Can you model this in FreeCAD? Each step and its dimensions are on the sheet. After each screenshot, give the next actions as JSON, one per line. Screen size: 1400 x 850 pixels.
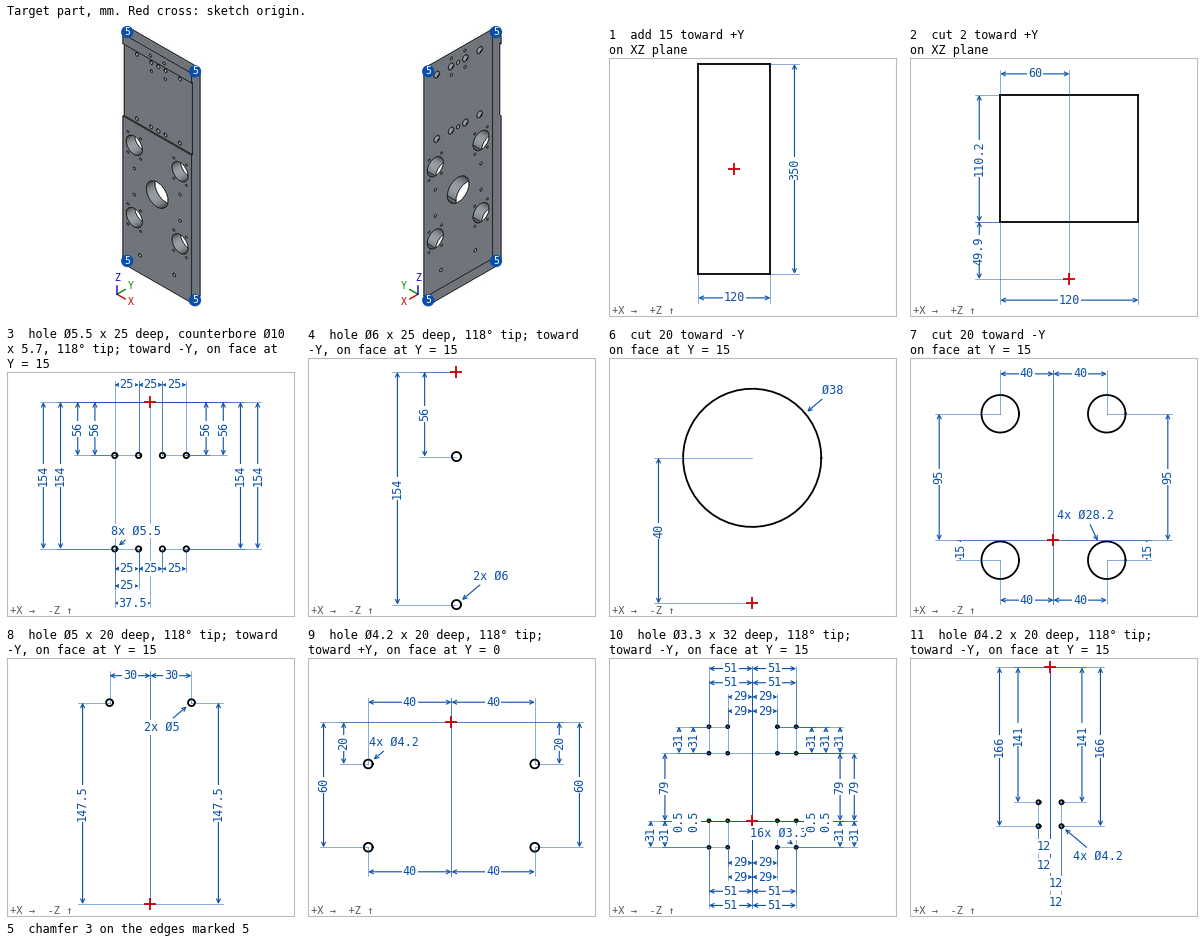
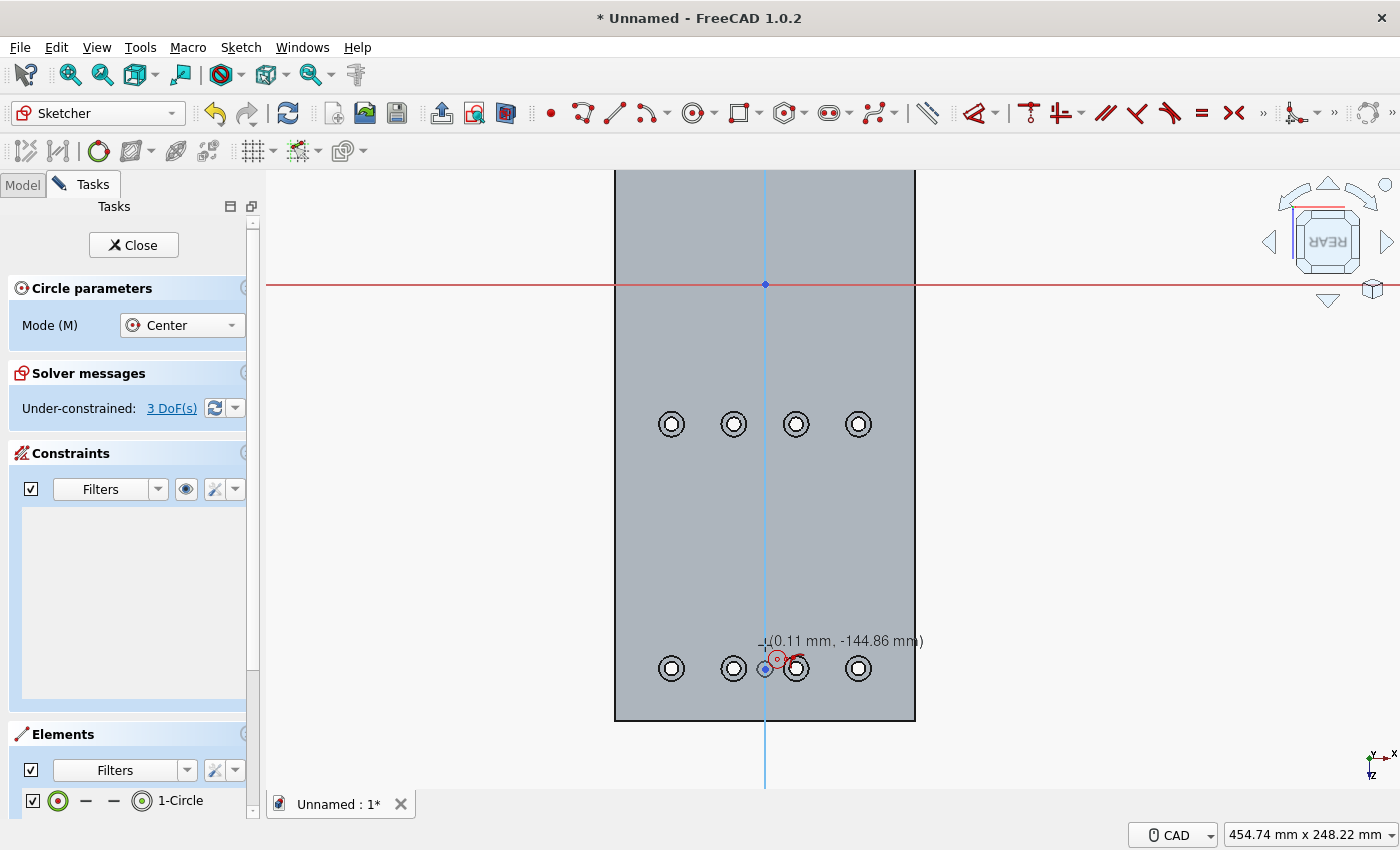
{"action": "scroll", "coordinate": [765, 424], "scroll_direction": "up", "scroll_amount": 6}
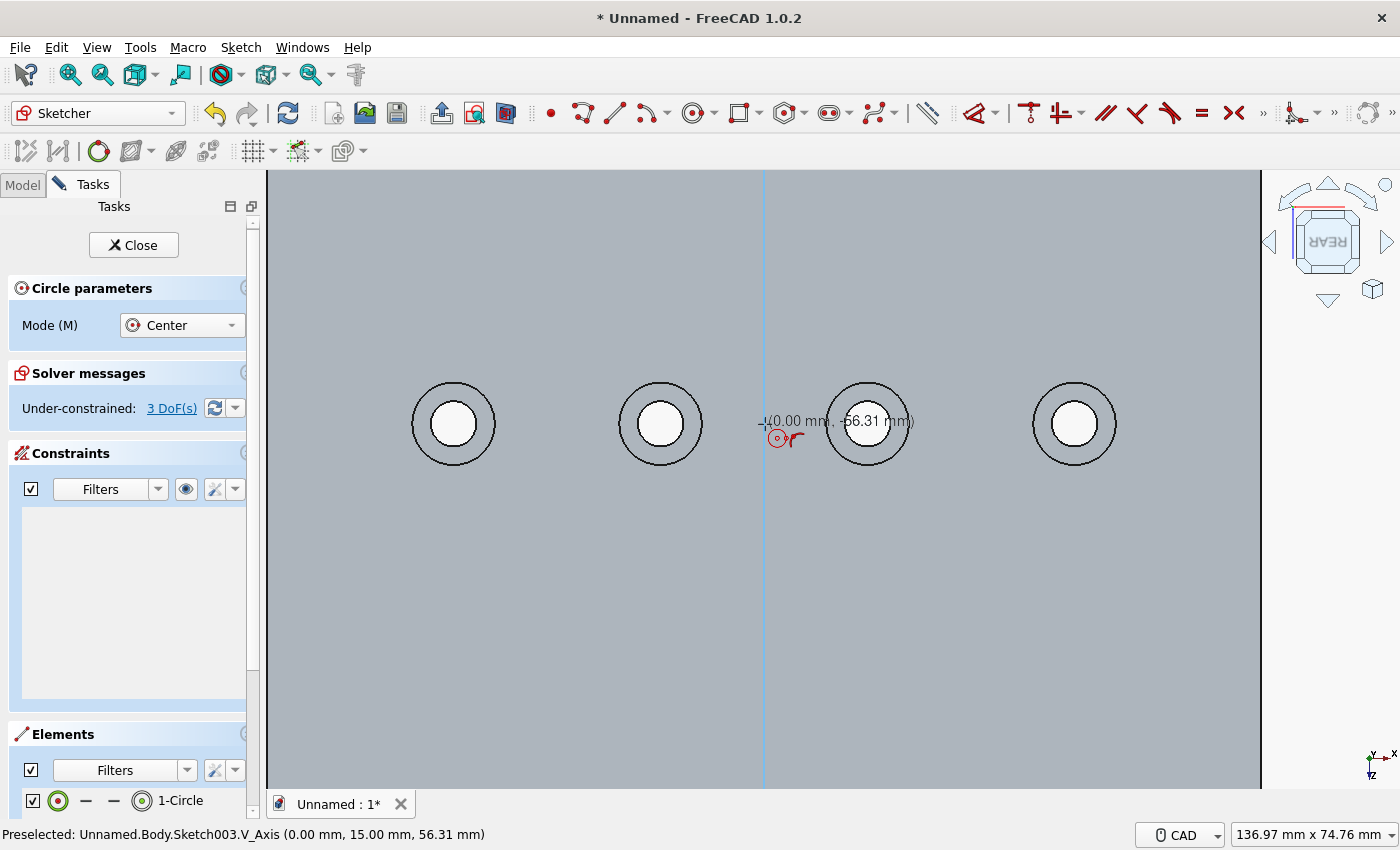
{"action": "left_click", "coordinate": [764, 424]}
{"action": "left_click", "coordinate": [782, 406]}
{"action": "key", "text": "Escape"}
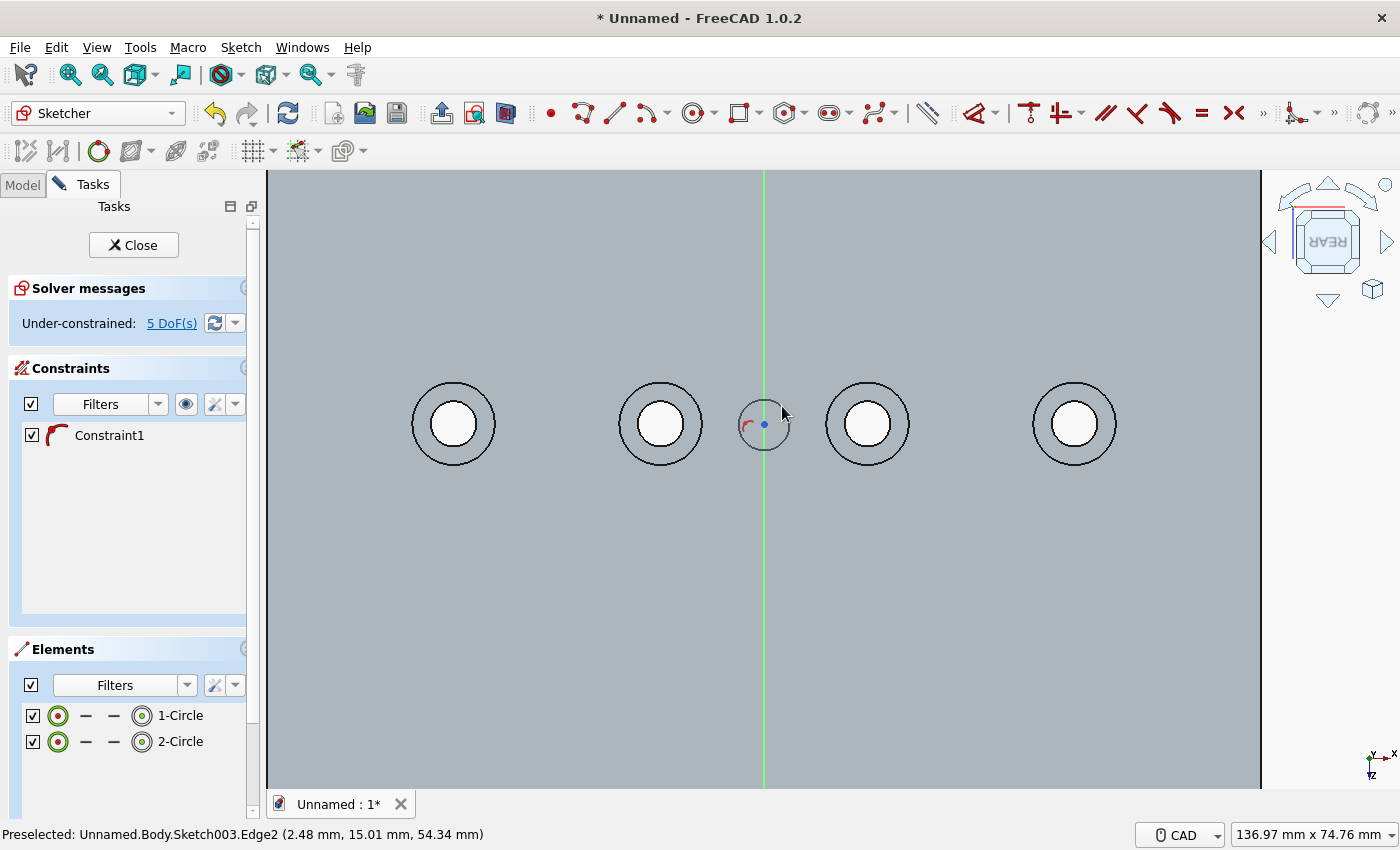
{"action": "scroll", "coordinate": [765, 423], "scroll_direction": "down", "scroll_amount": 6}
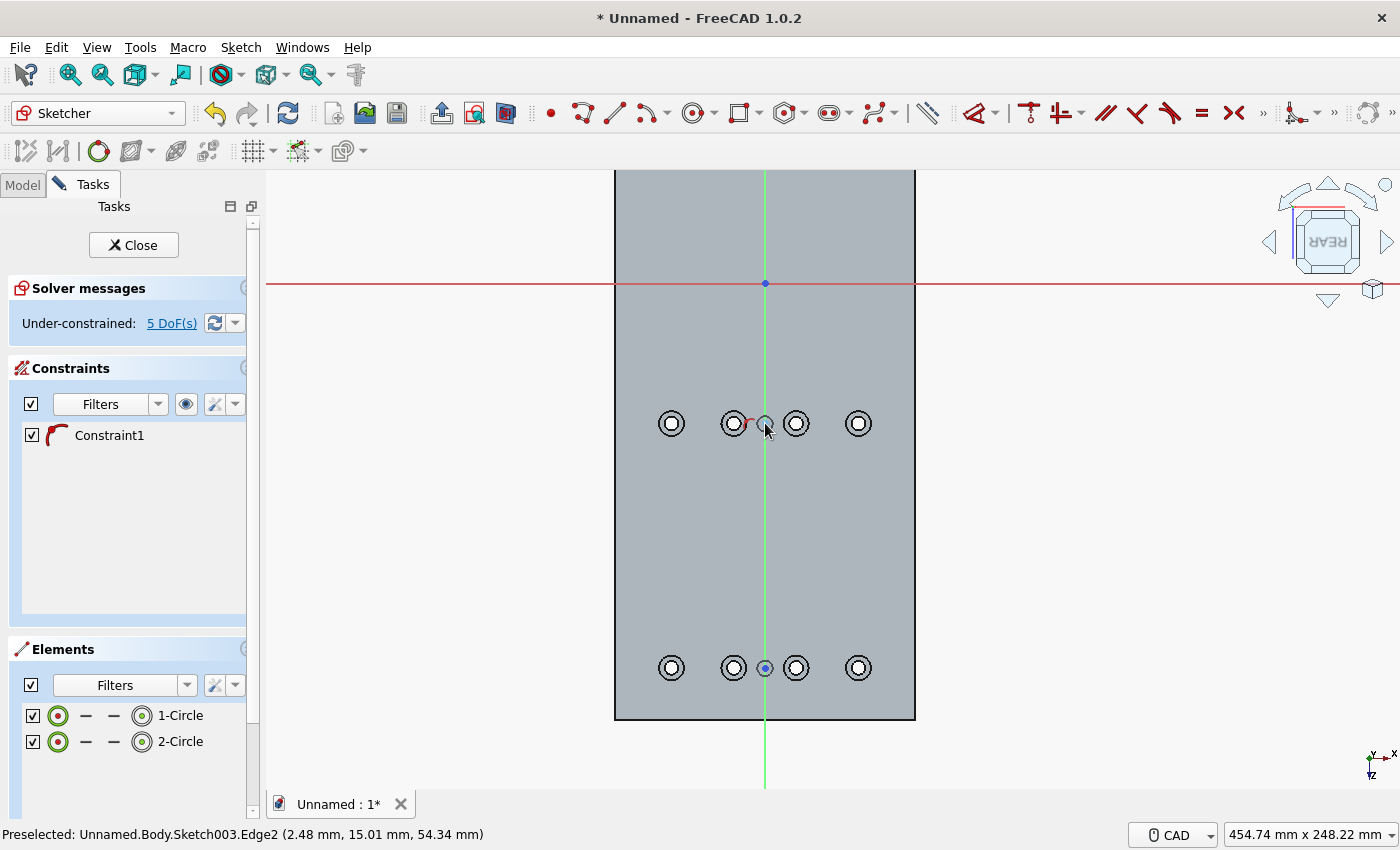
{"action": "scroll", "coordinate": [770, 663], "scroll_direction": "up", "scroll_amount": 5}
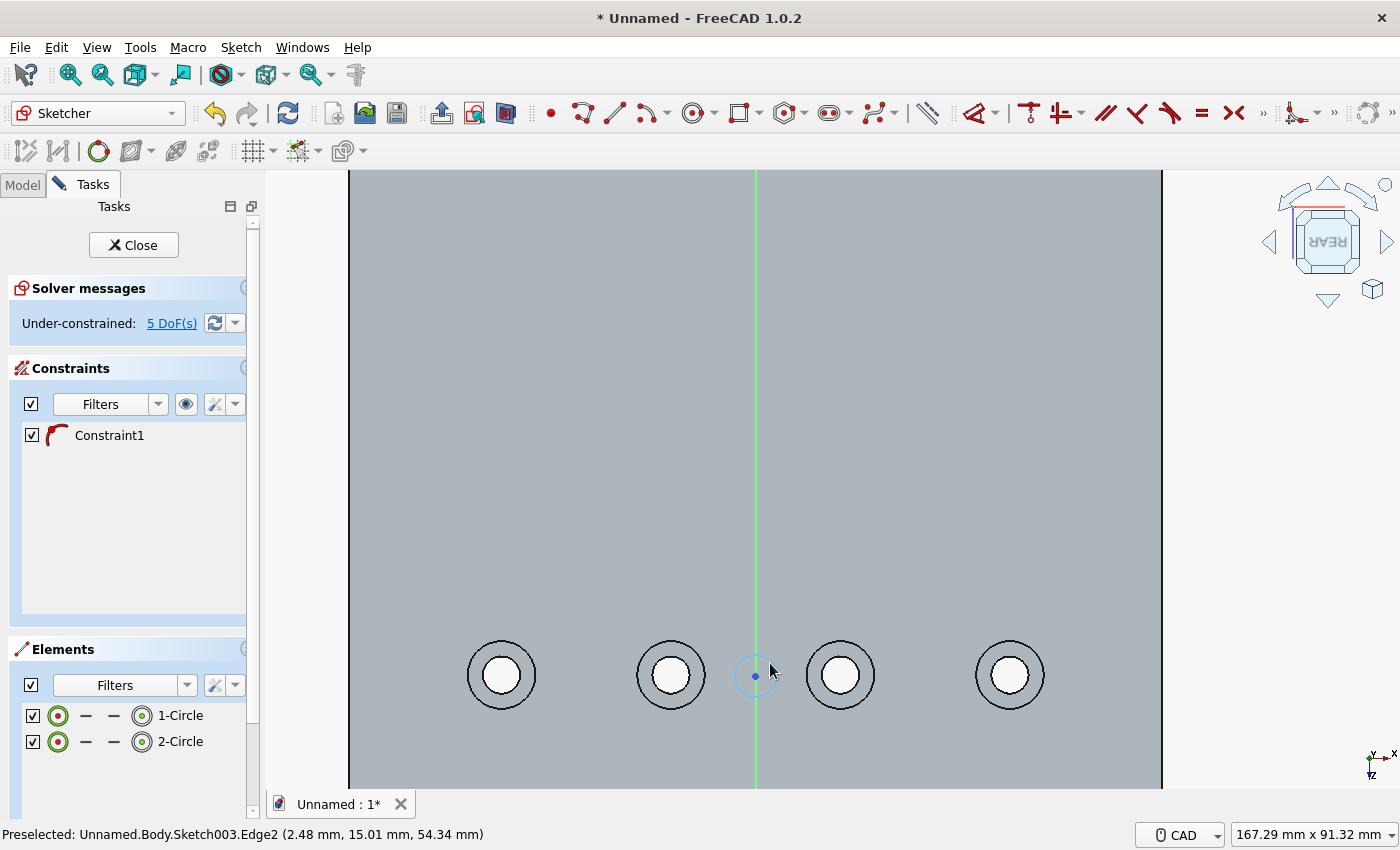
{"action": "left_click", "coordinate": [770, 661]}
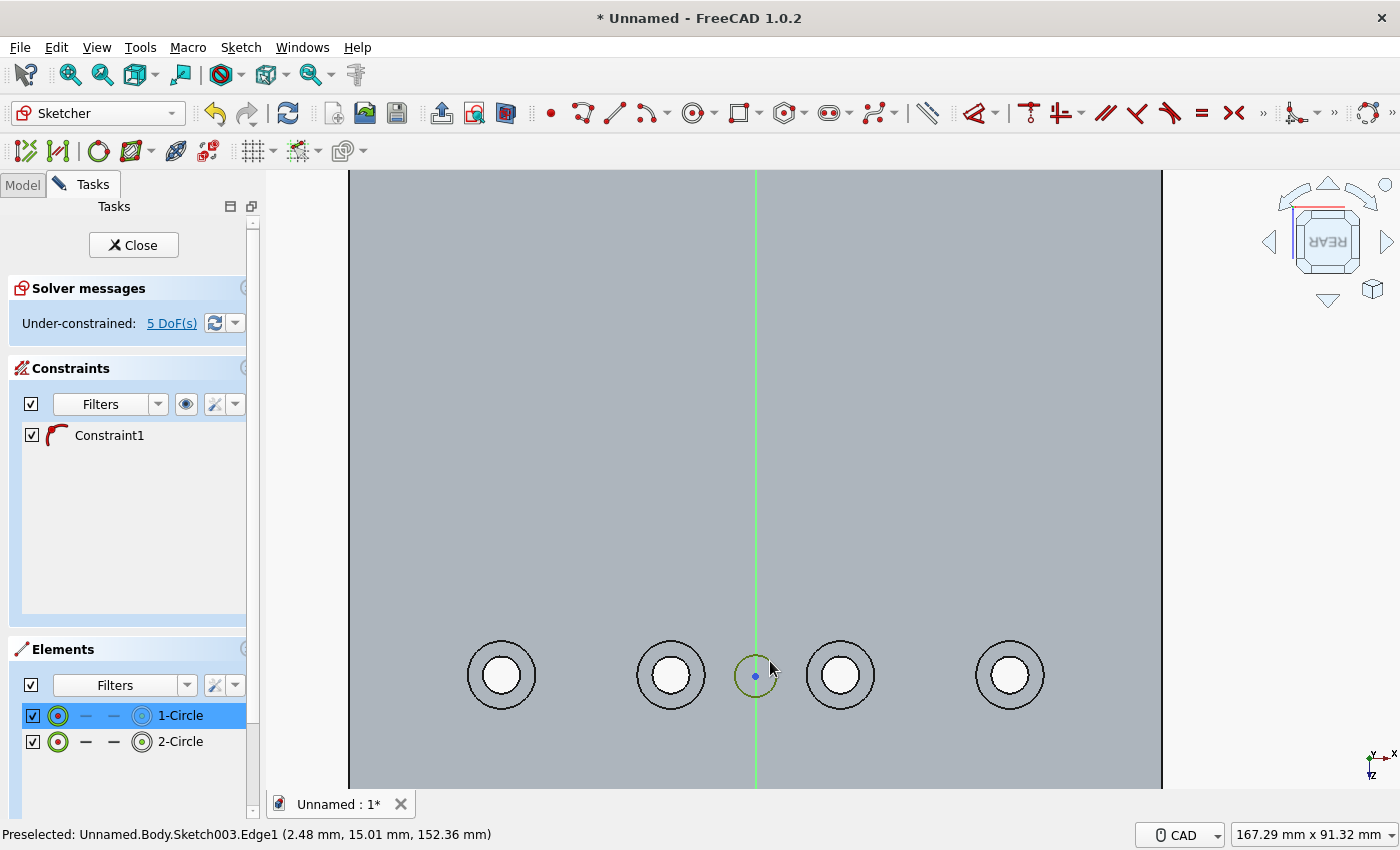
{"action": "scroll", "coordinate": [770, 664], "scroll_direction": "down", "scroll_amount": 5}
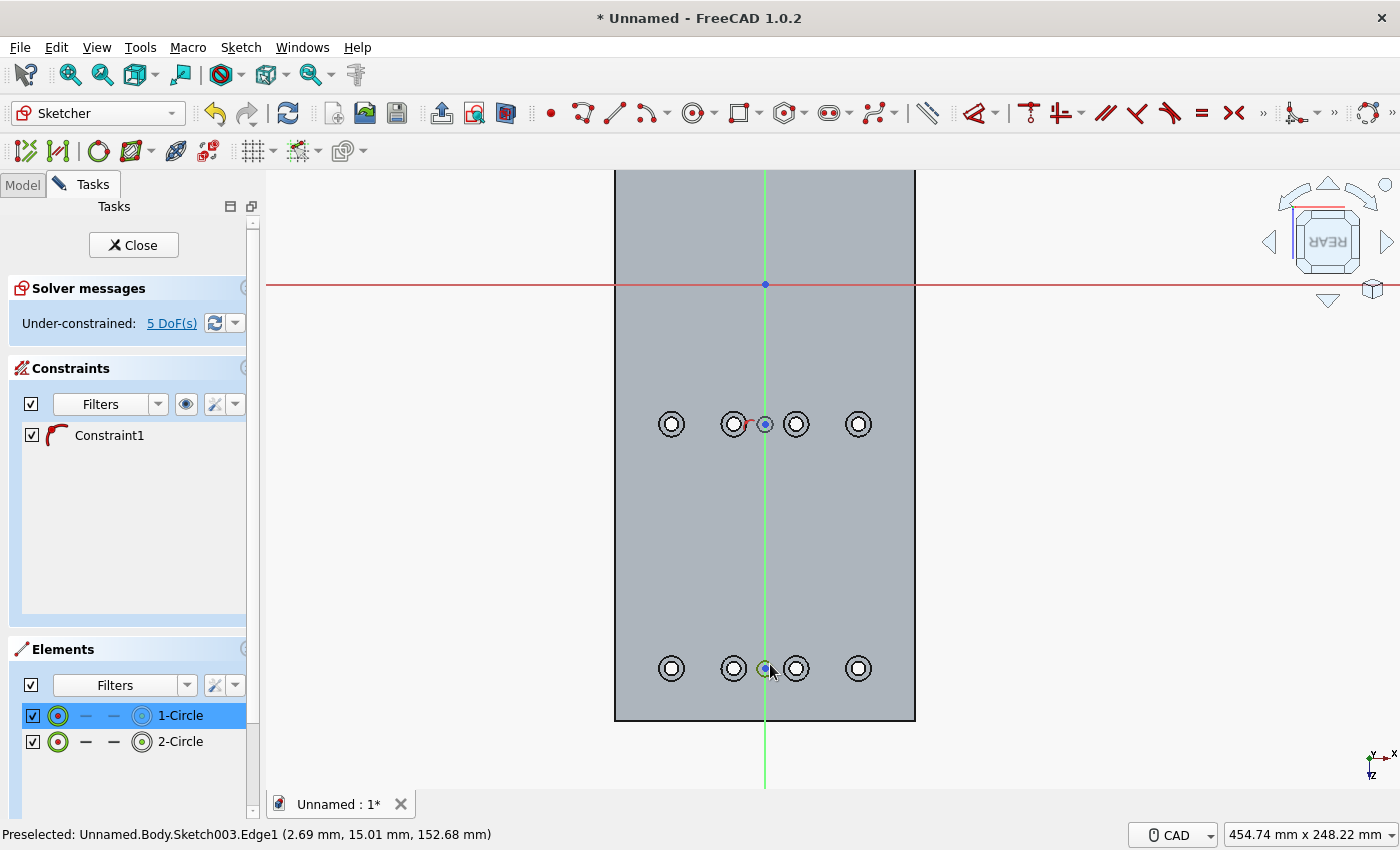
{"action": "scroll", "coordinate": [770, 419], "scroll_direction": "up", "scroll_amount": 5}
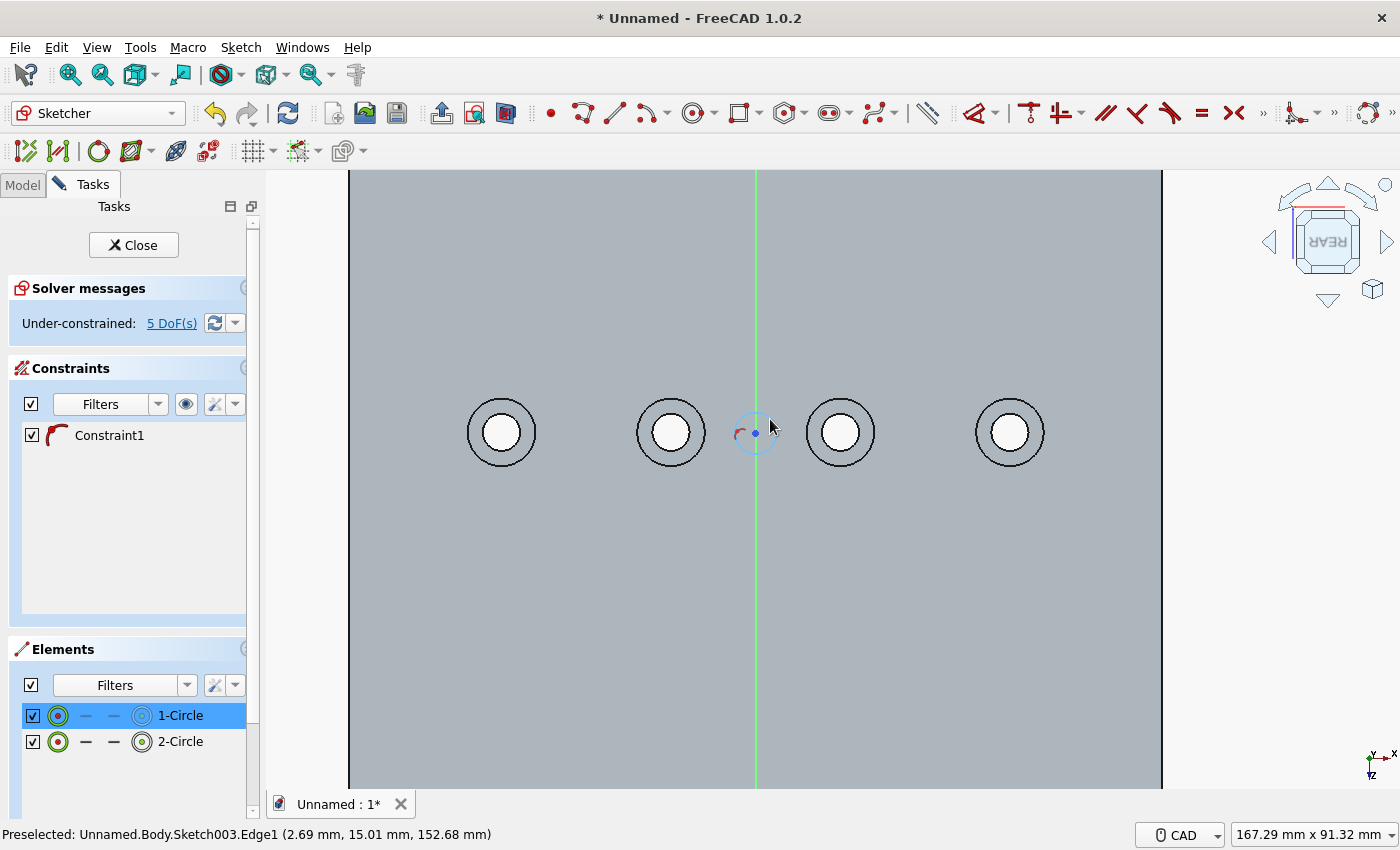
{"action": "left_click", "coordinate": [770, 419]}